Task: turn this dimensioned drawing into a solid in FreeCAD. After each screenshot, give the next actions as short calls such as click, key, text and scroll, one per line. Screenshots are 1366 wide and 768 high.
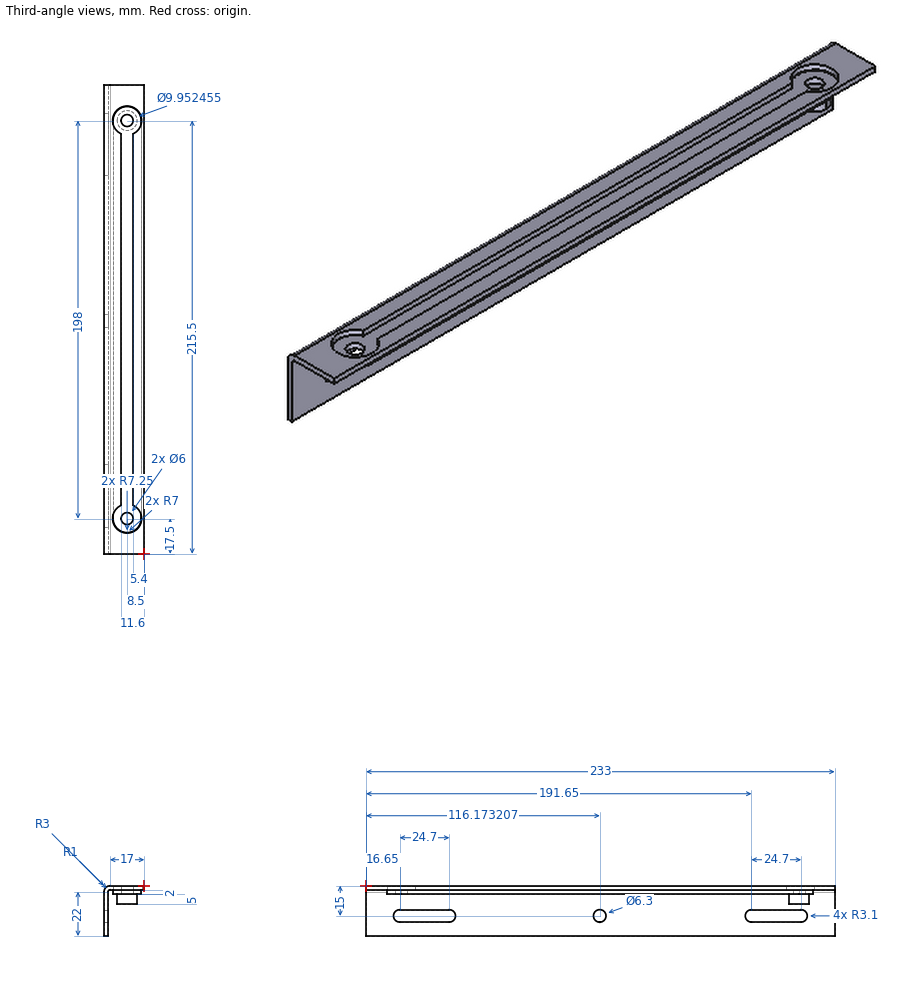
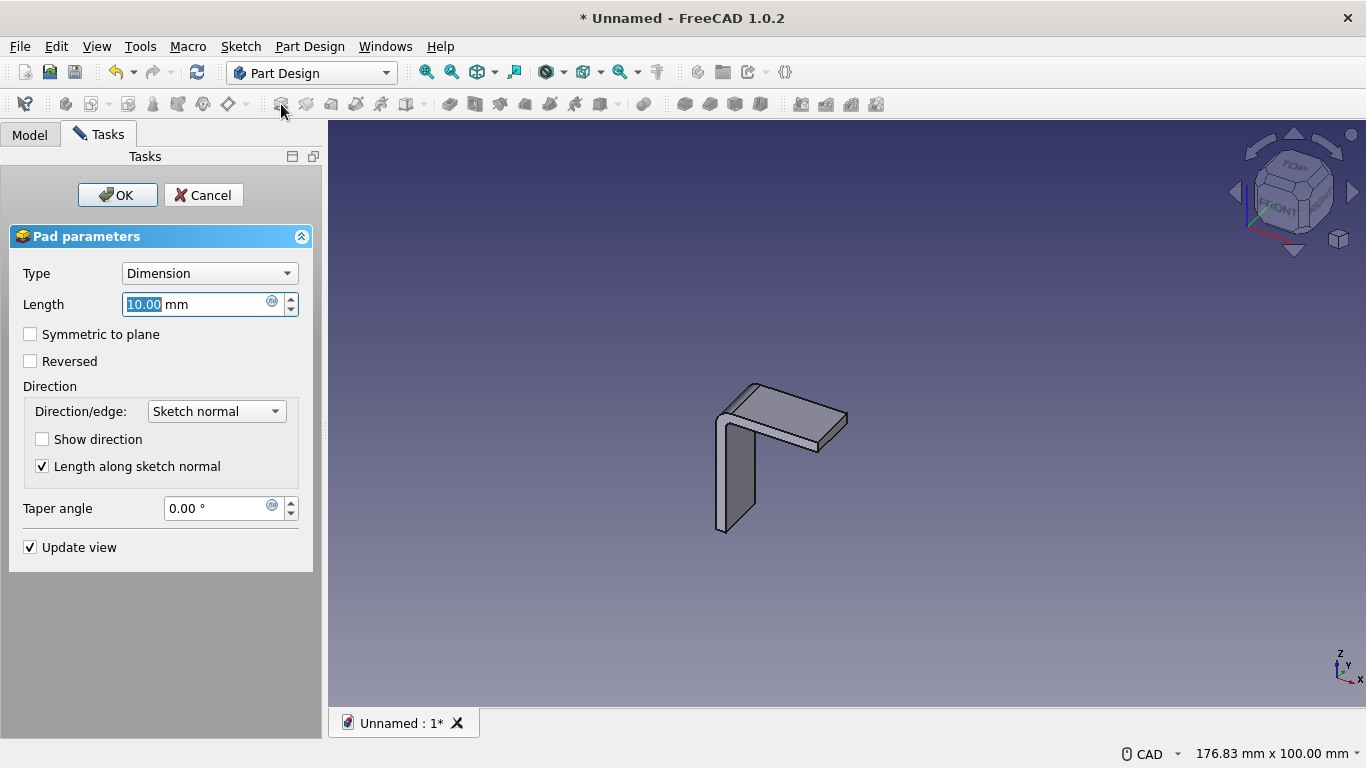
text(233)
key(Tab)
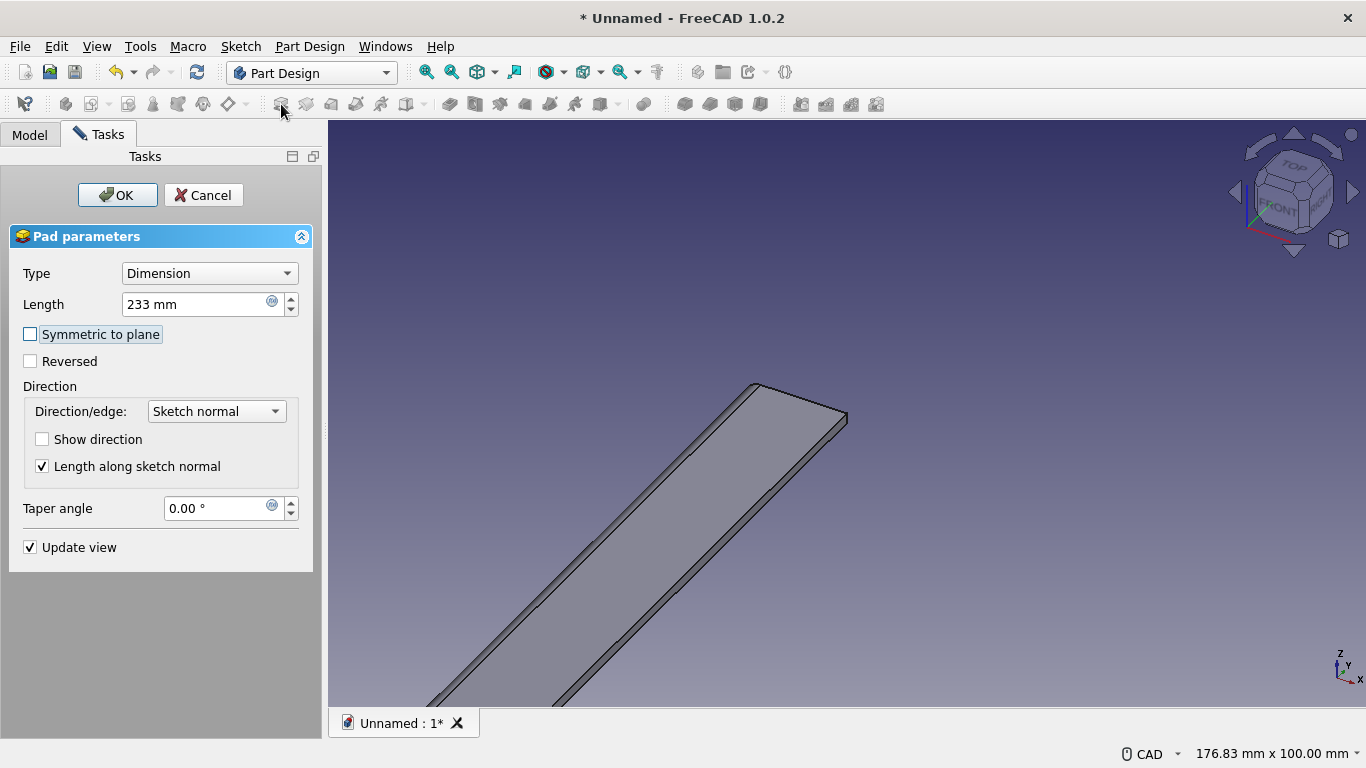
click(31, 361)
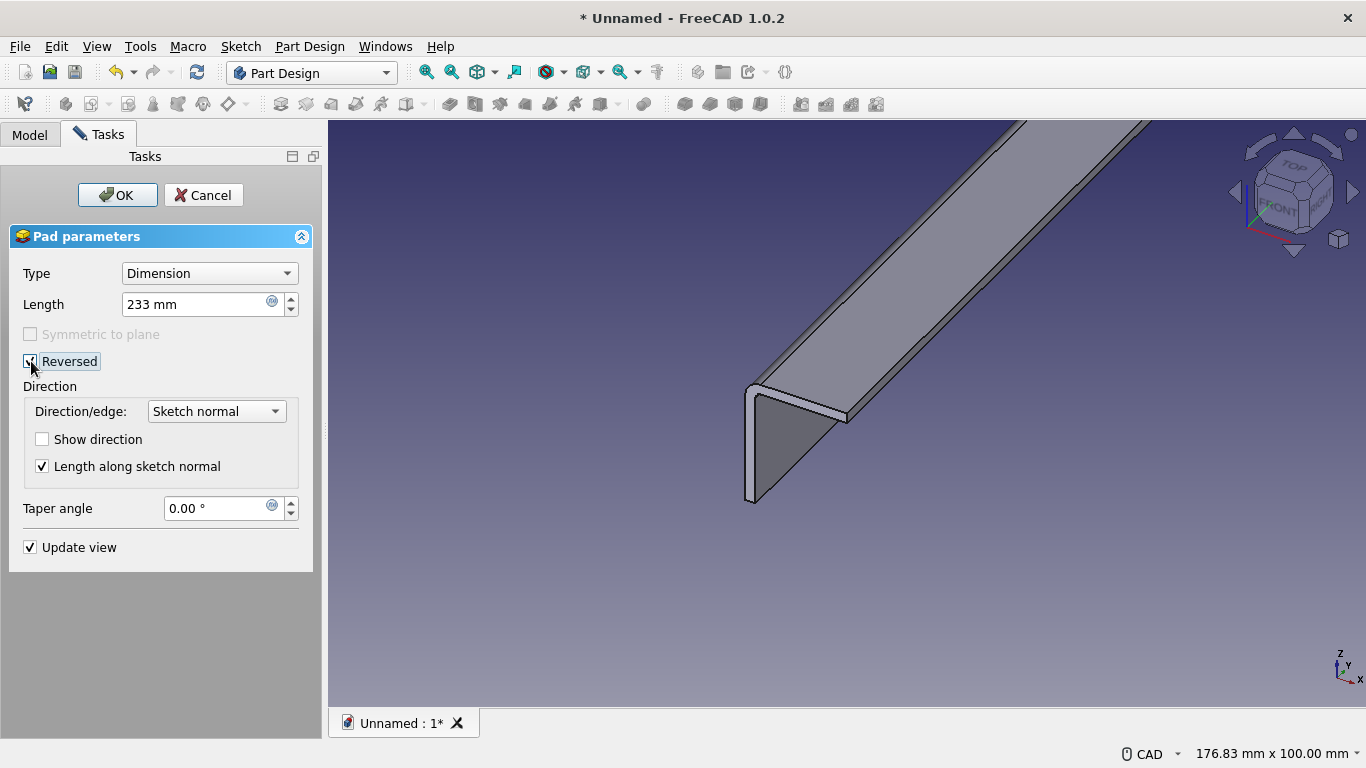
click(118, 195)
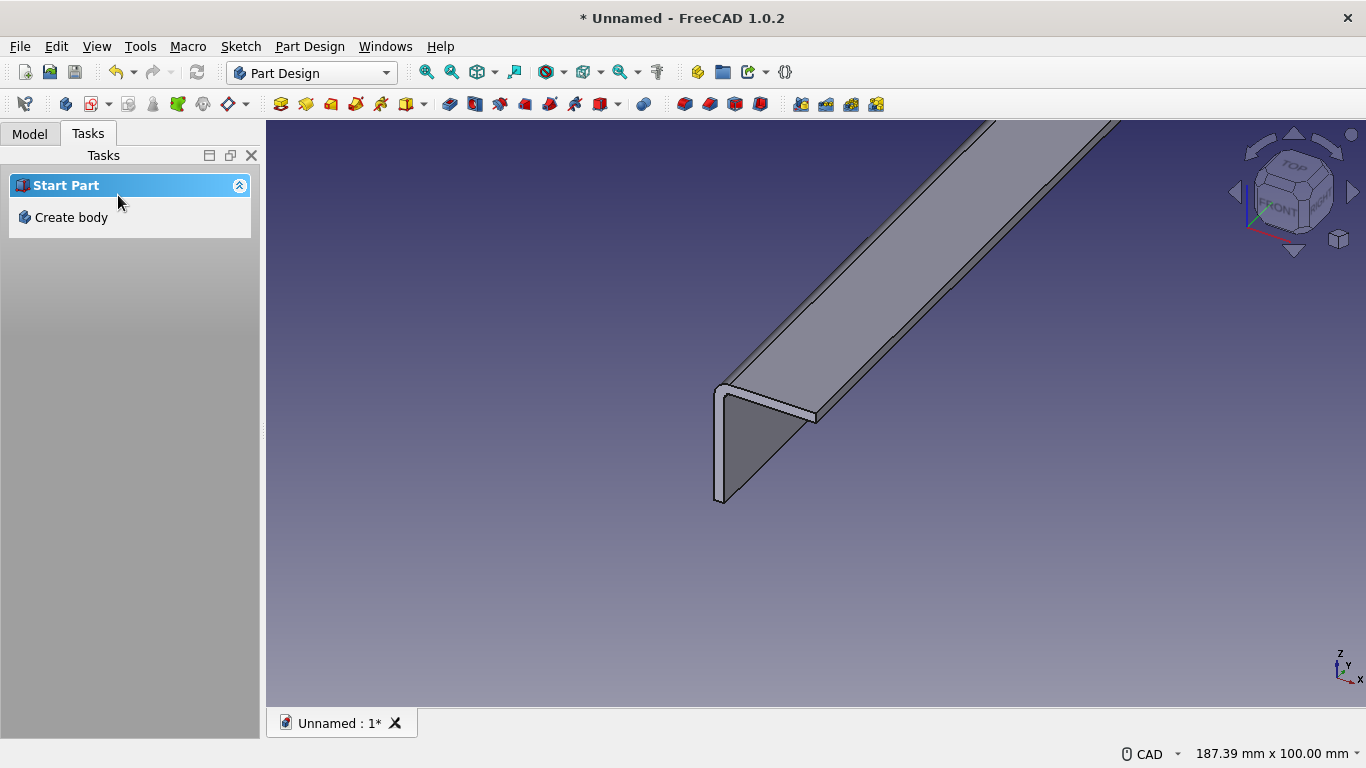
click(427, 72)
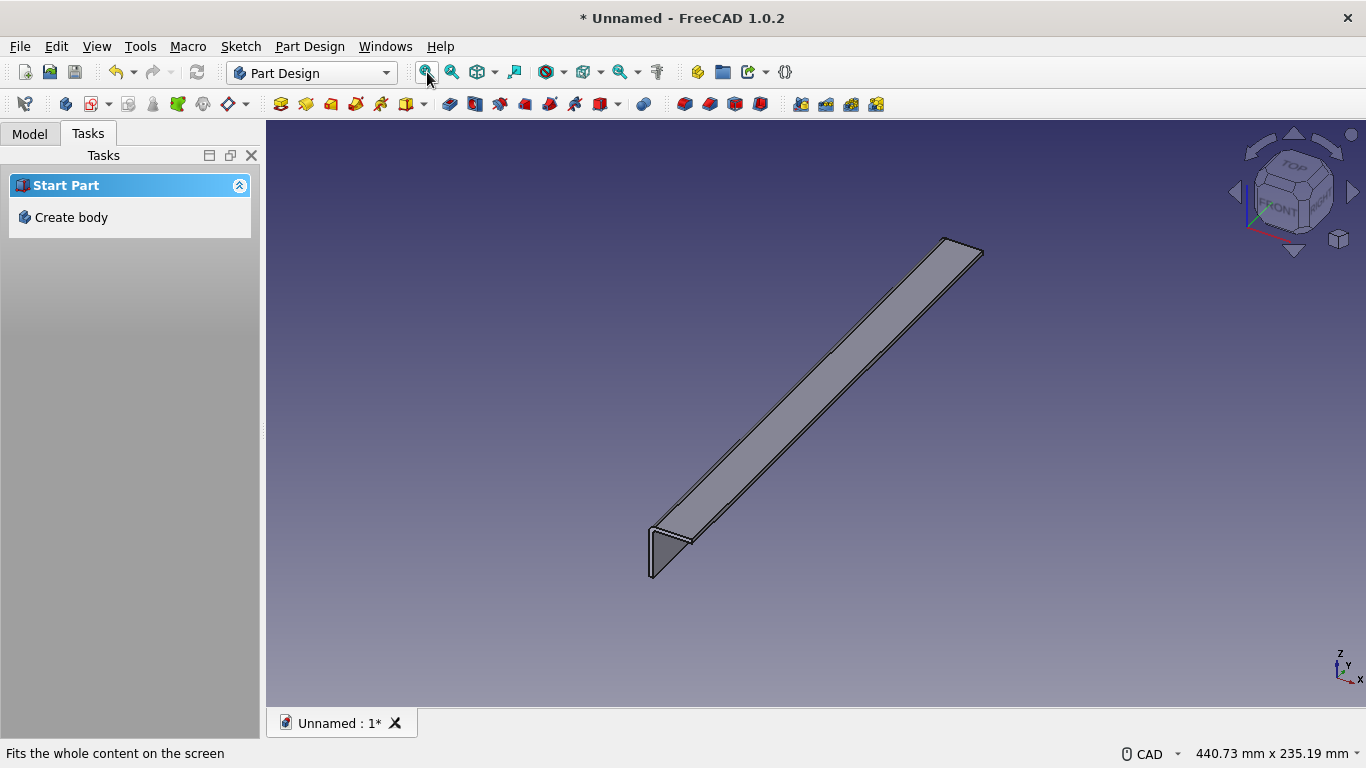
click(30, 134)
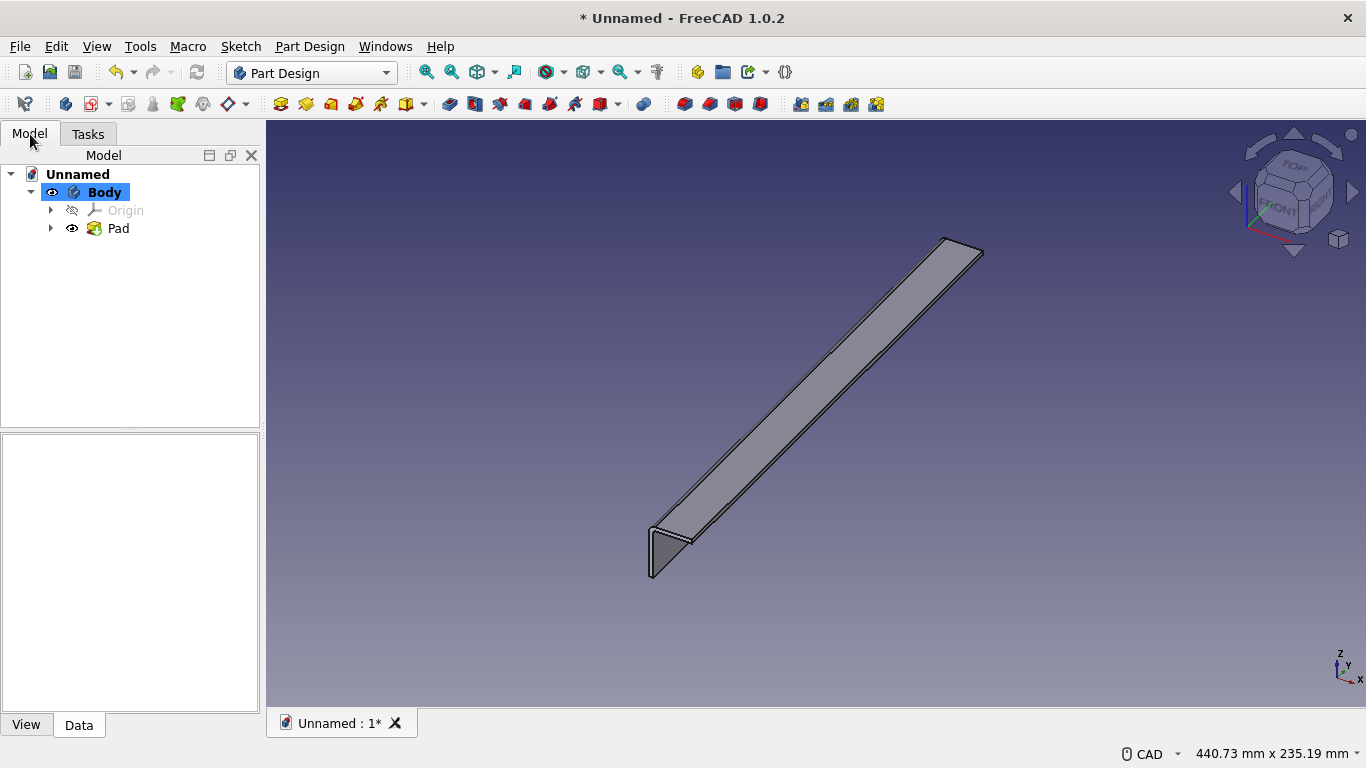
click(51, 210)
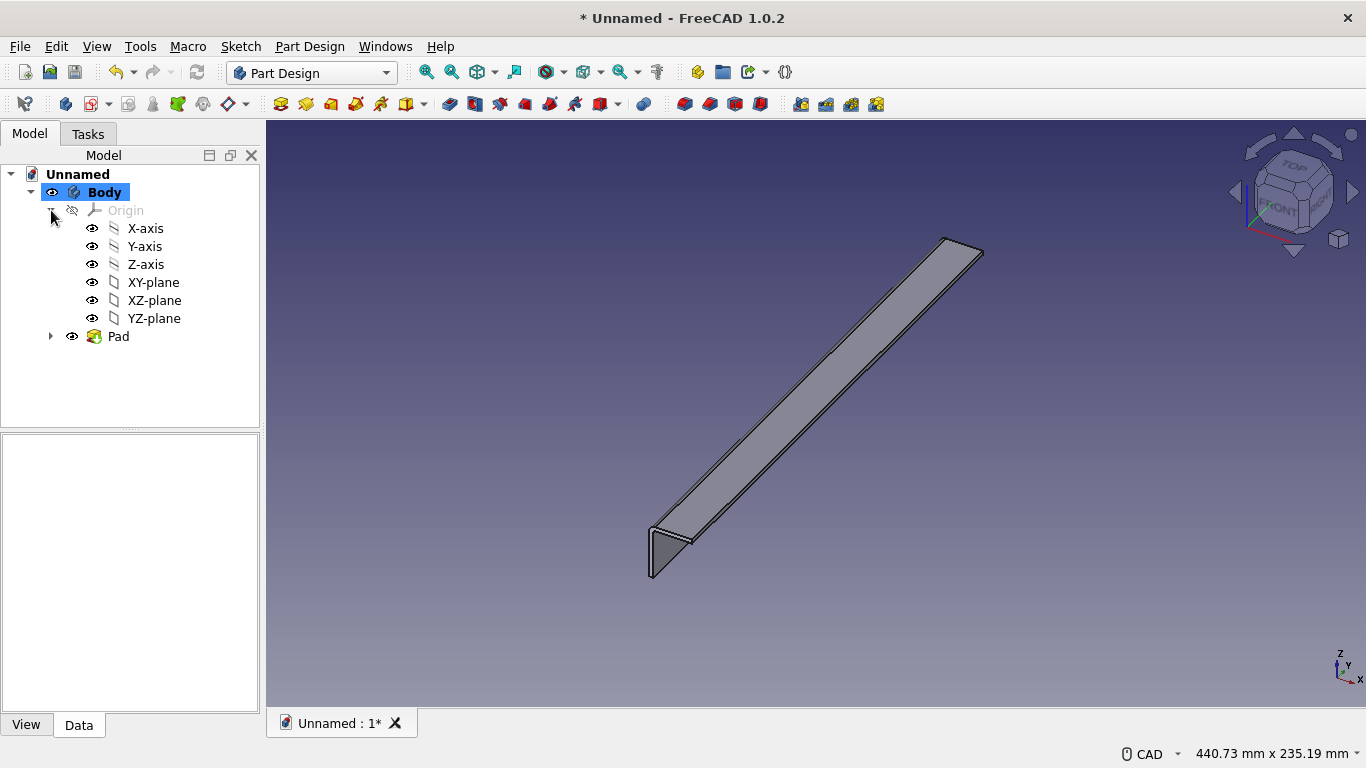
click(137, 318)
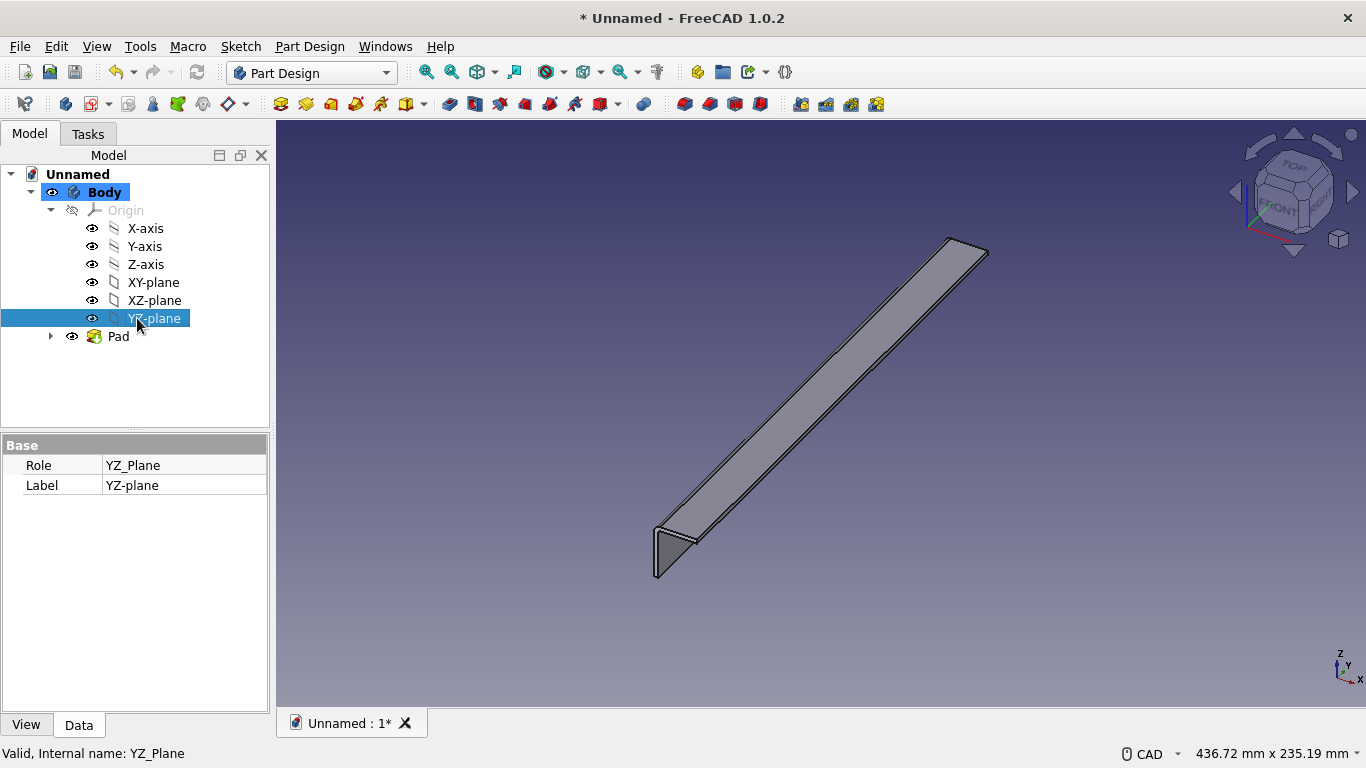
click(228, 104)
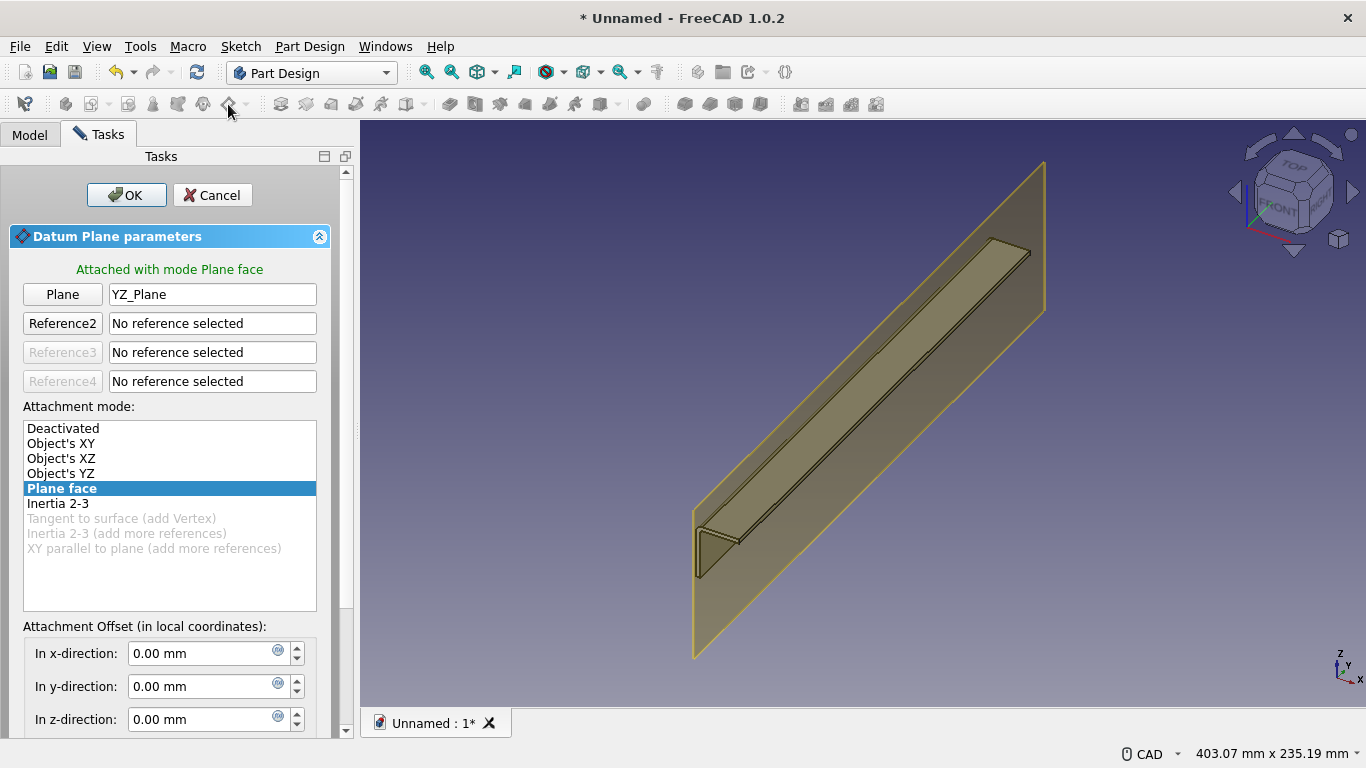
triple_click(210, 720)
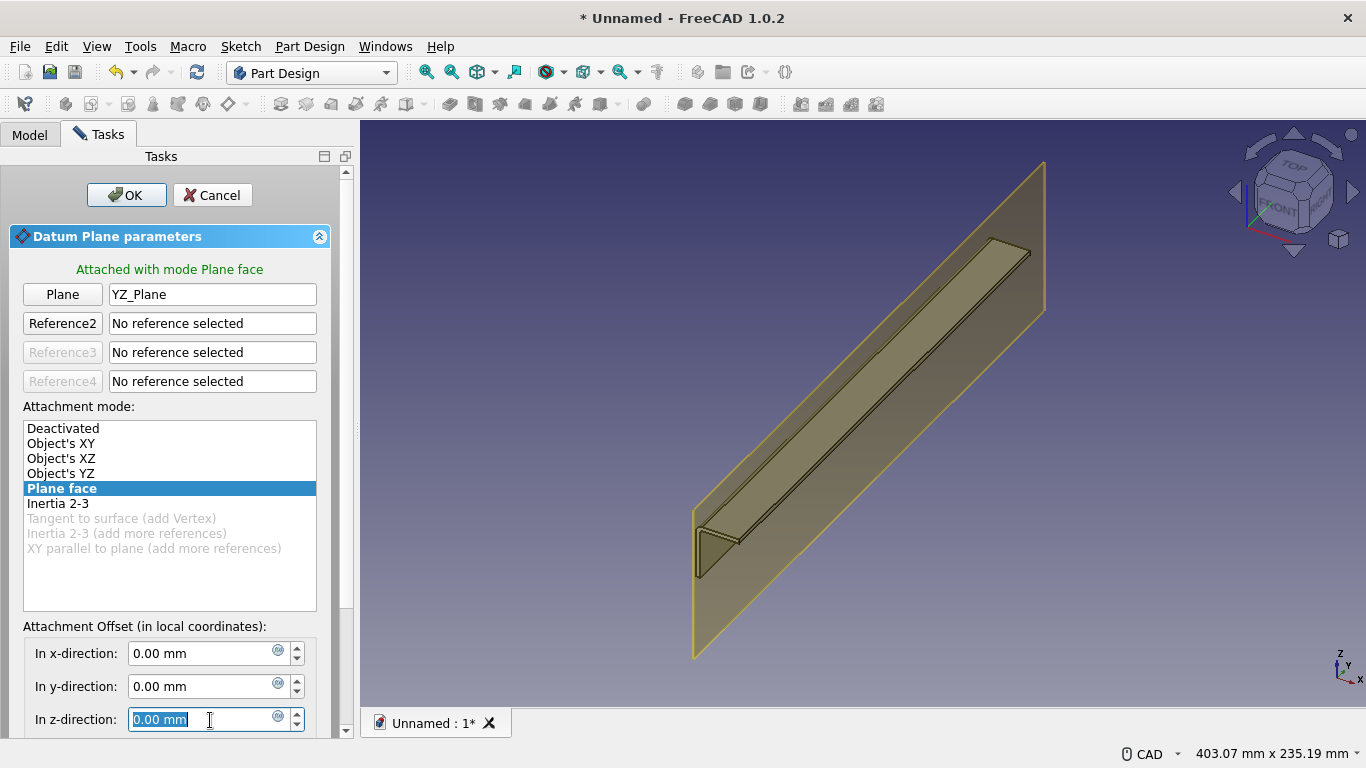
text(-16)
key(Tab)